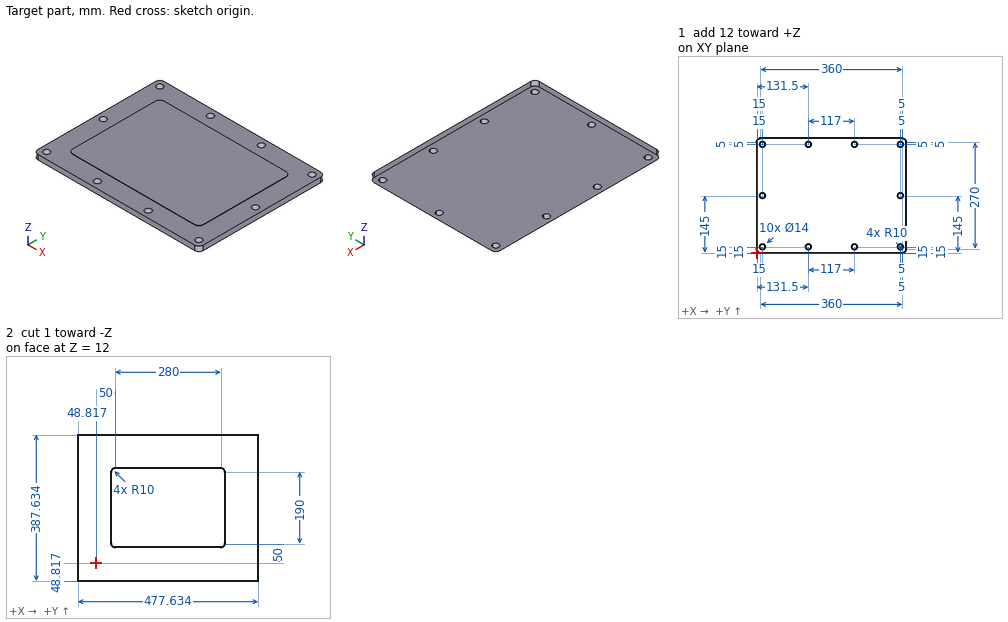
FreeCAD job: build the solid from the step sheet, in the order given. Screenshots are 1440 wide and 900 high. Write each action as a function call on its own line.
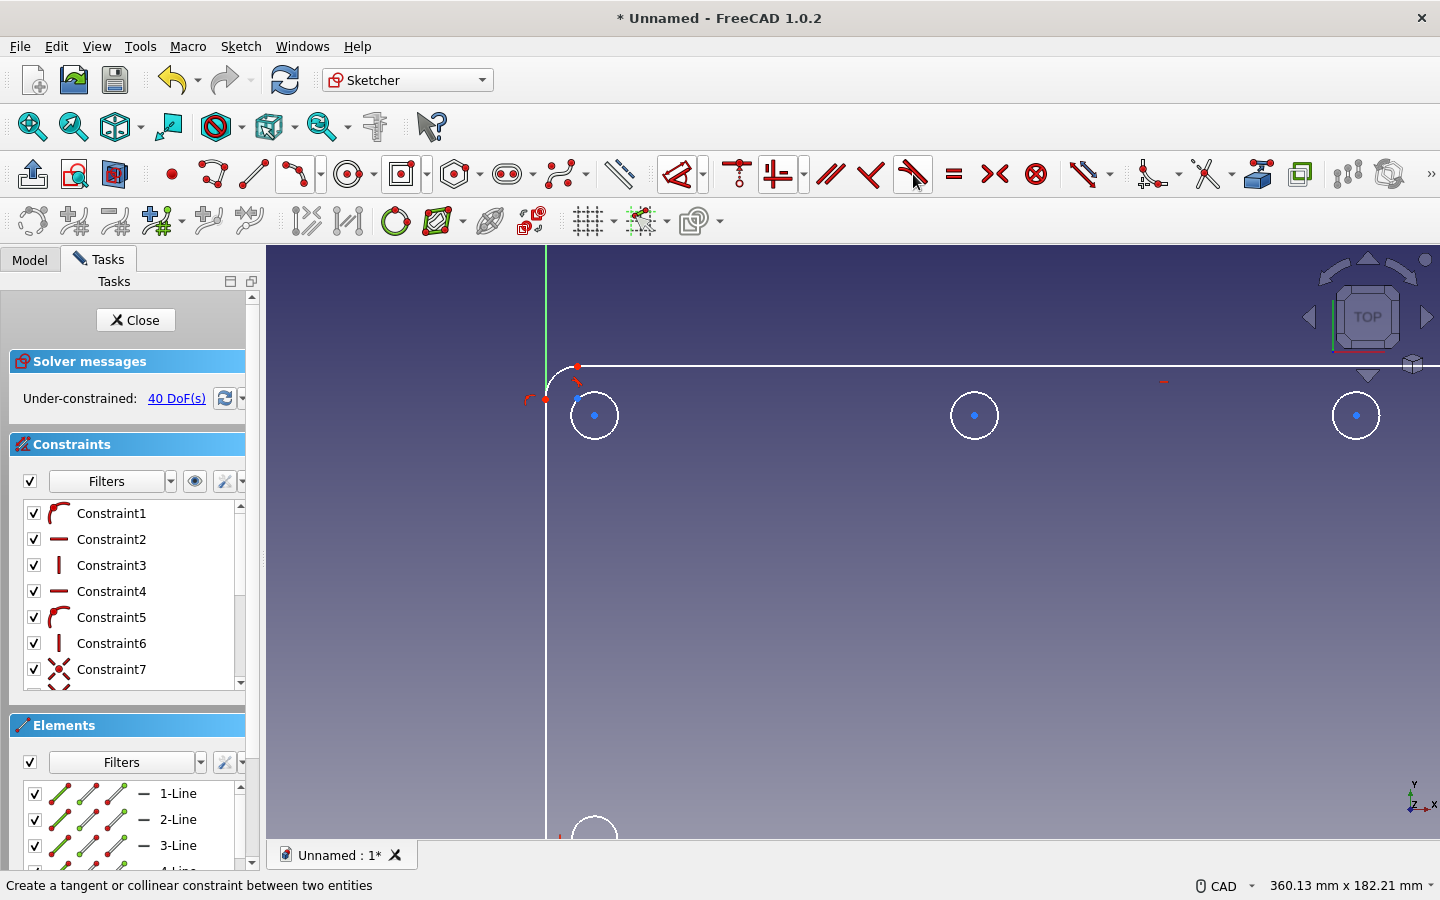
click(546, 664)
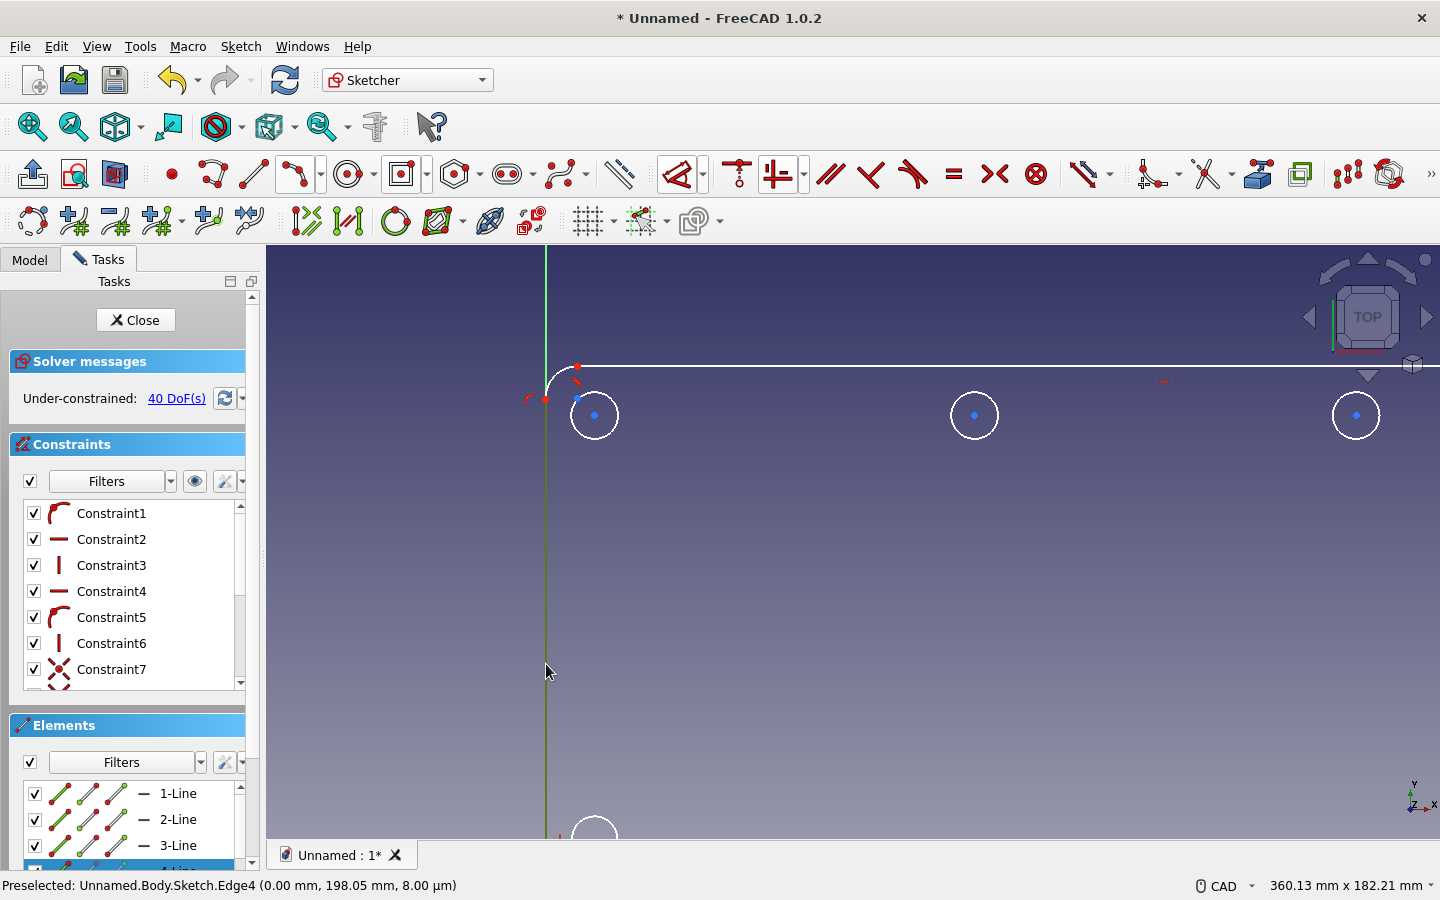
click(563, 370)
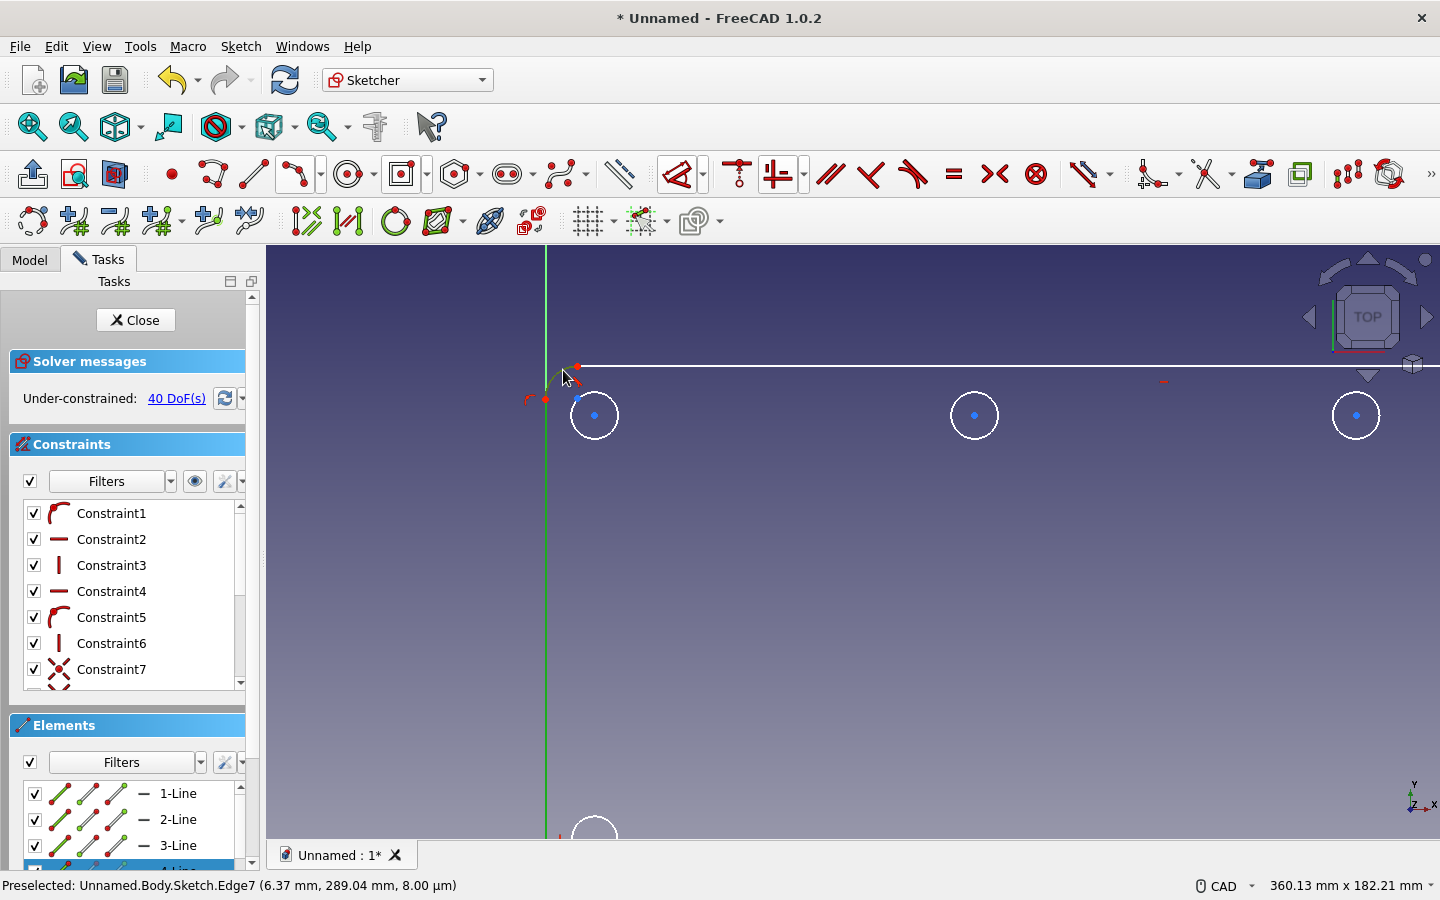
click(913, 174)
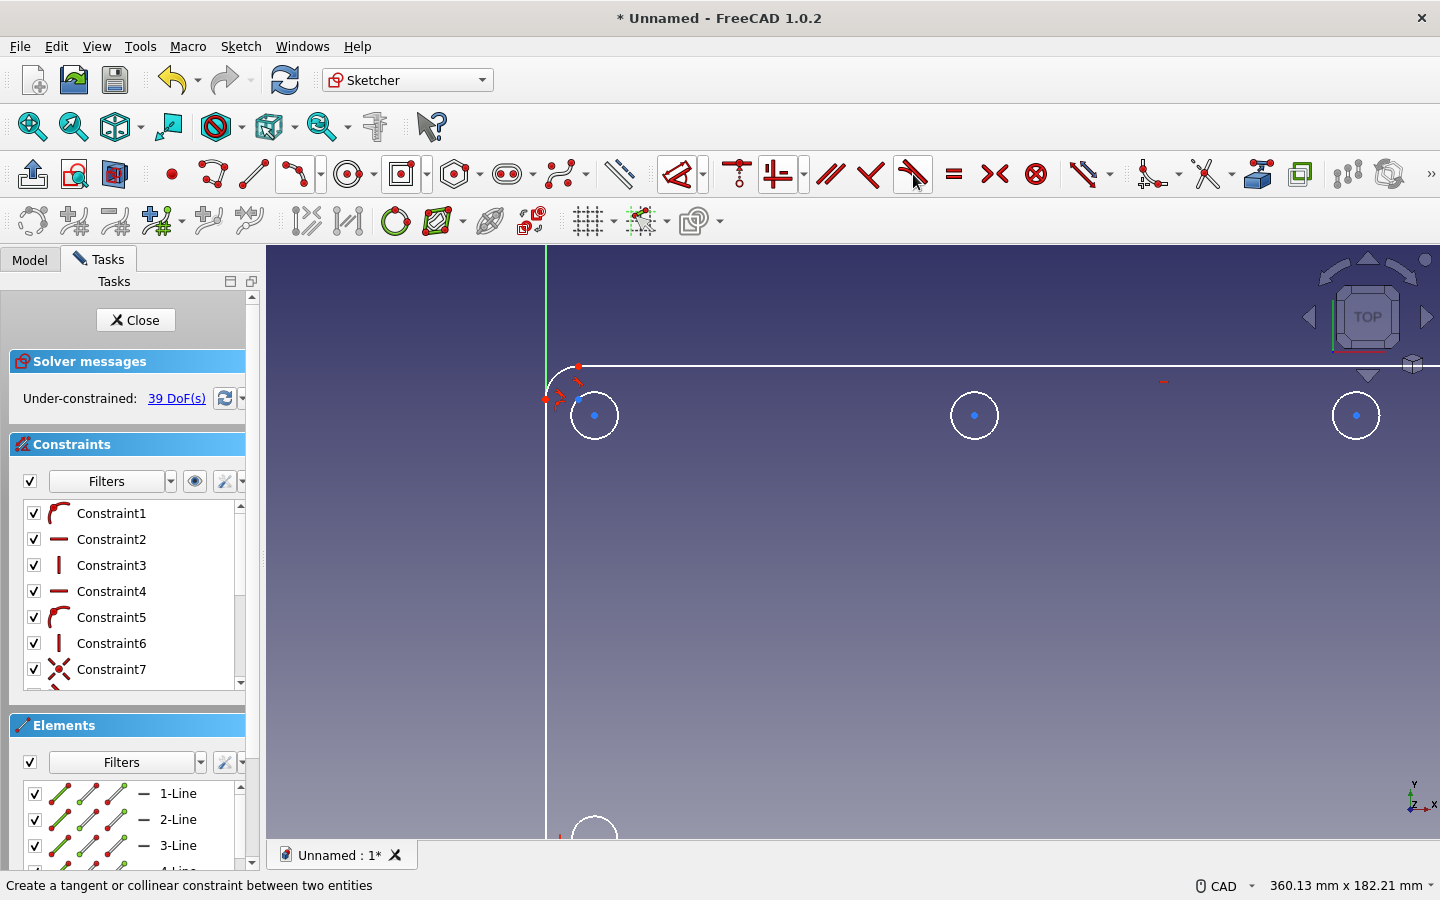
click(546, 664)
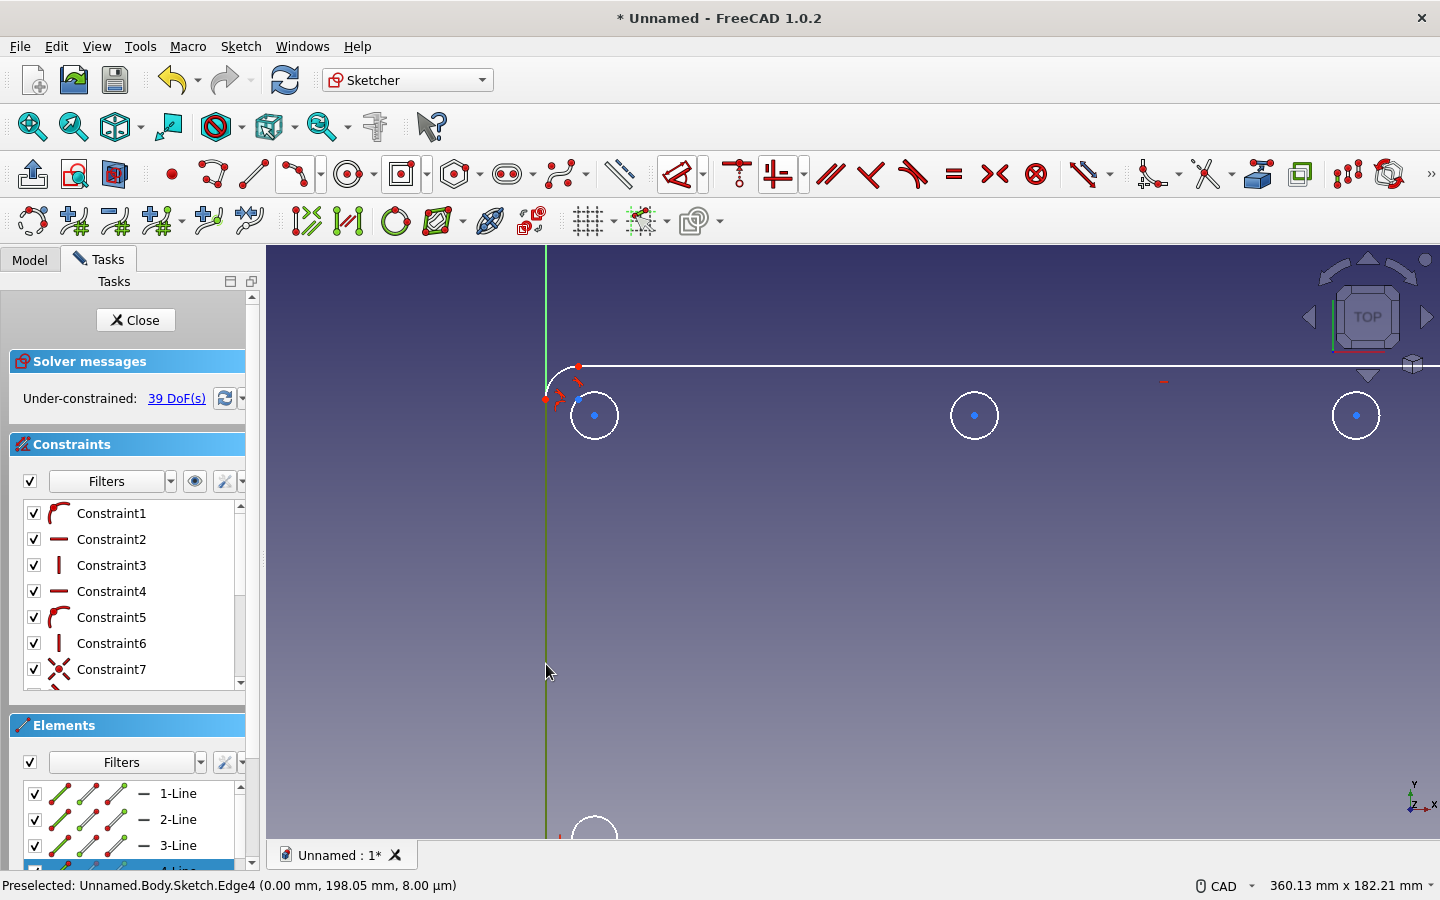
scroll(563, 370, down, 5)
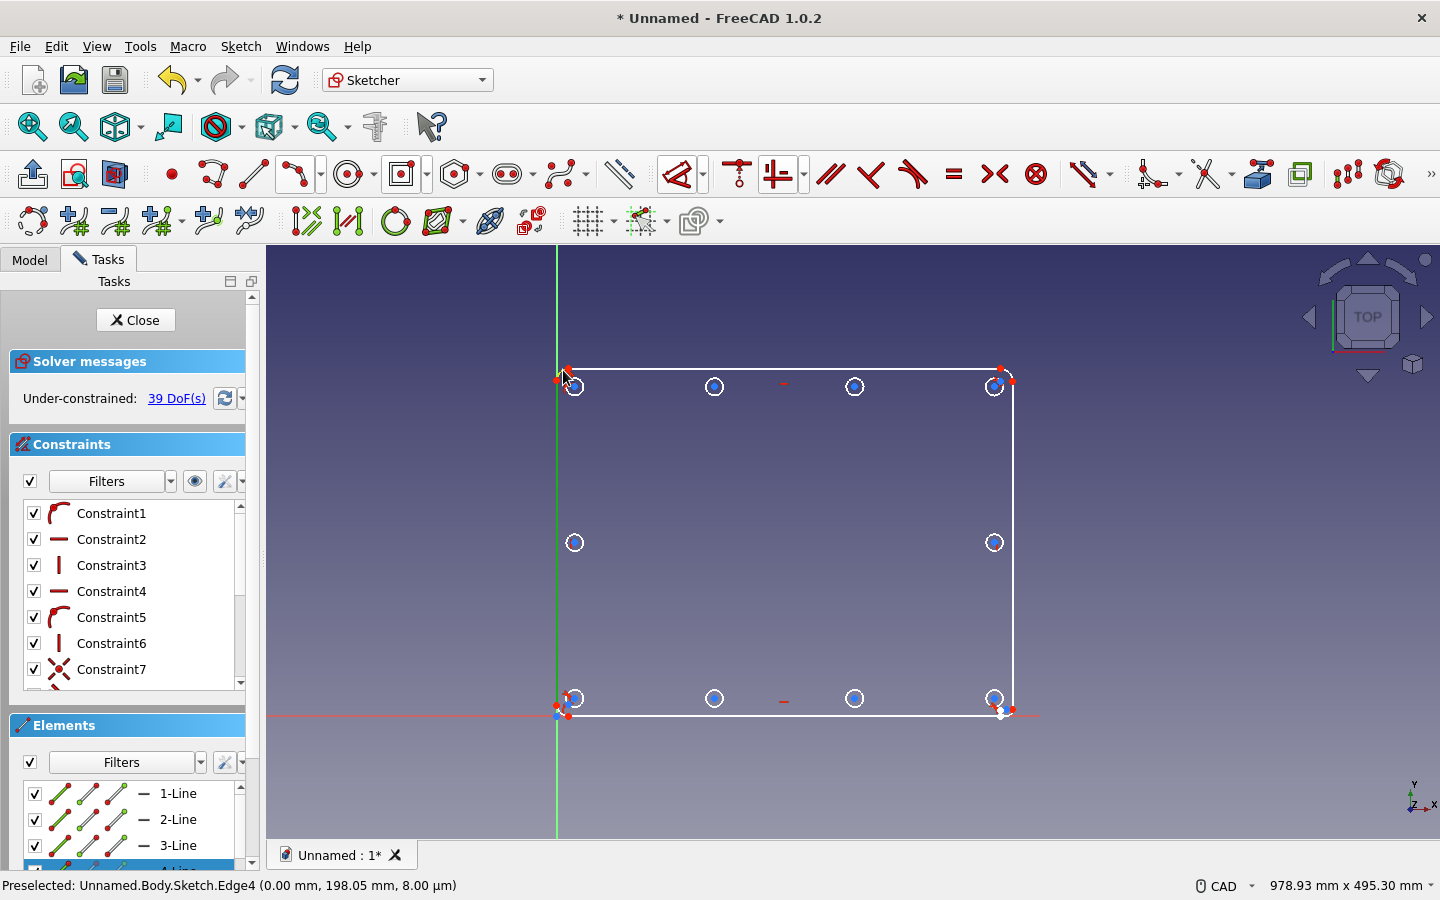
scroll(564, 715, up, 5)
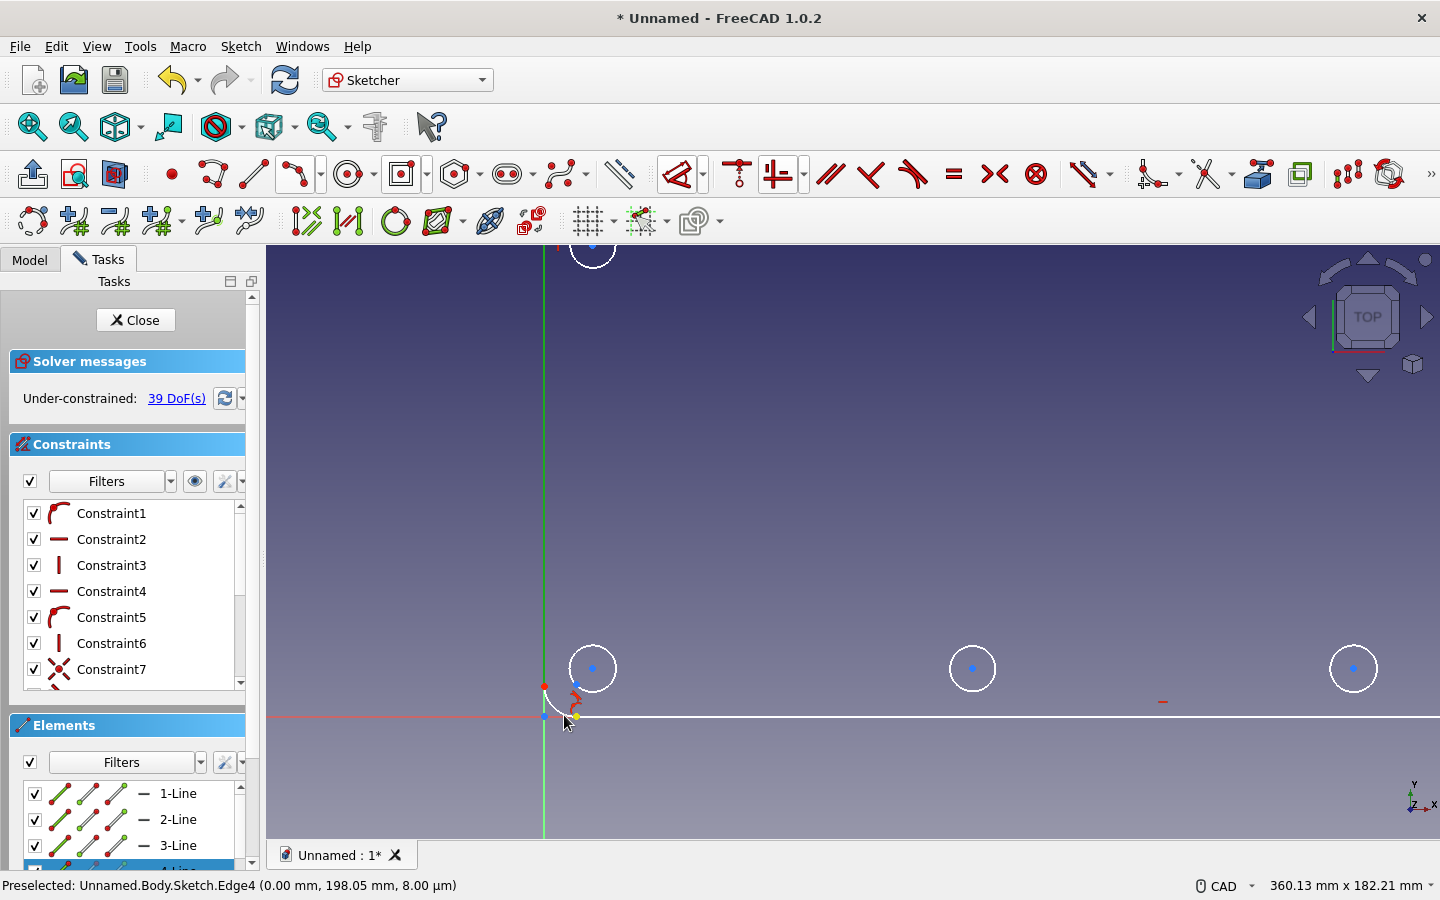
click(562, 714)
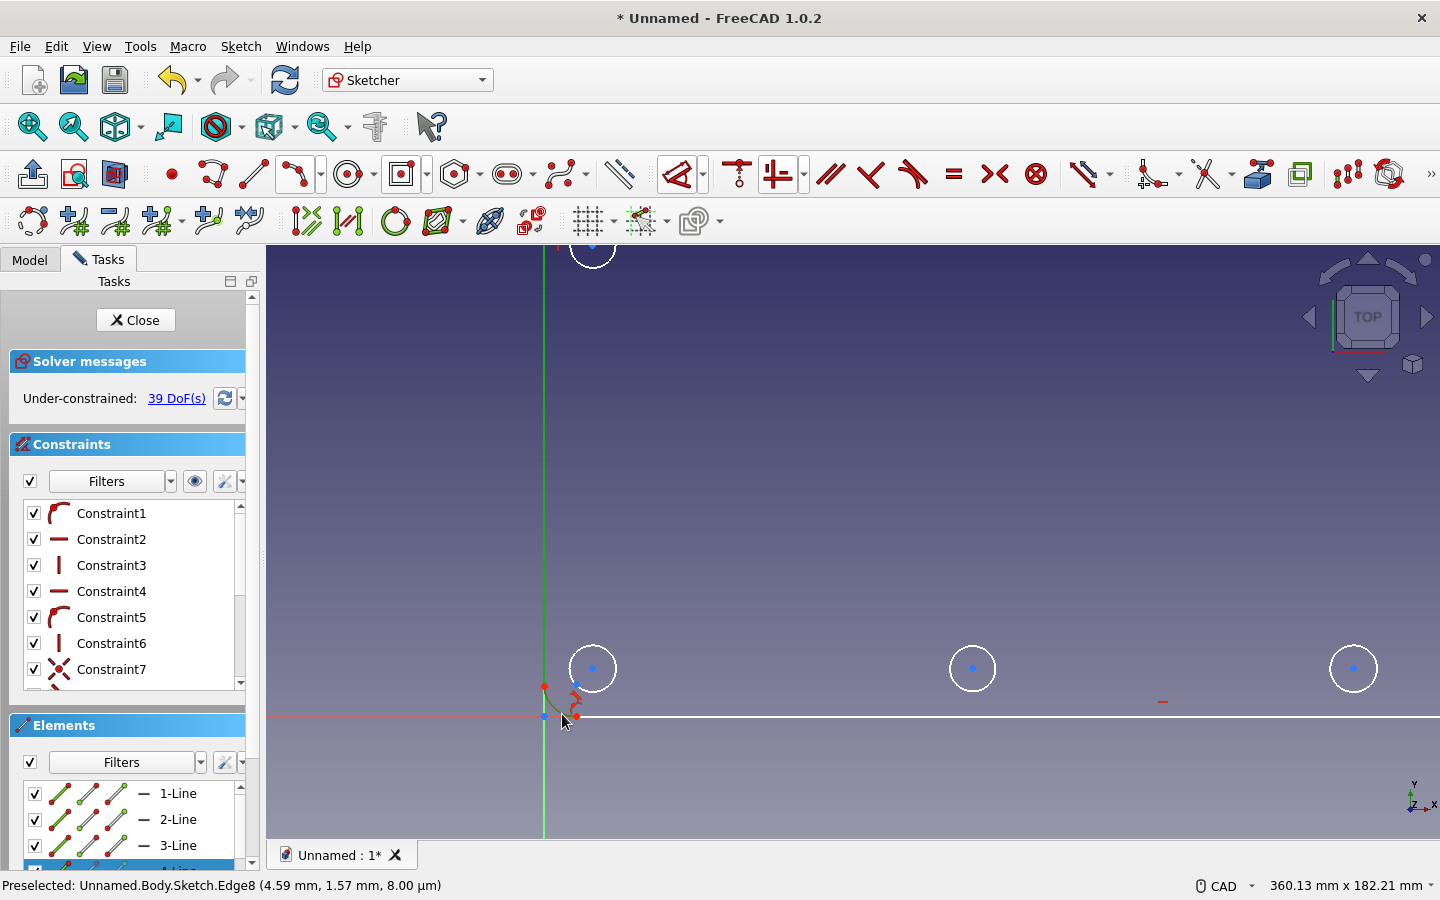
click(913, 174)